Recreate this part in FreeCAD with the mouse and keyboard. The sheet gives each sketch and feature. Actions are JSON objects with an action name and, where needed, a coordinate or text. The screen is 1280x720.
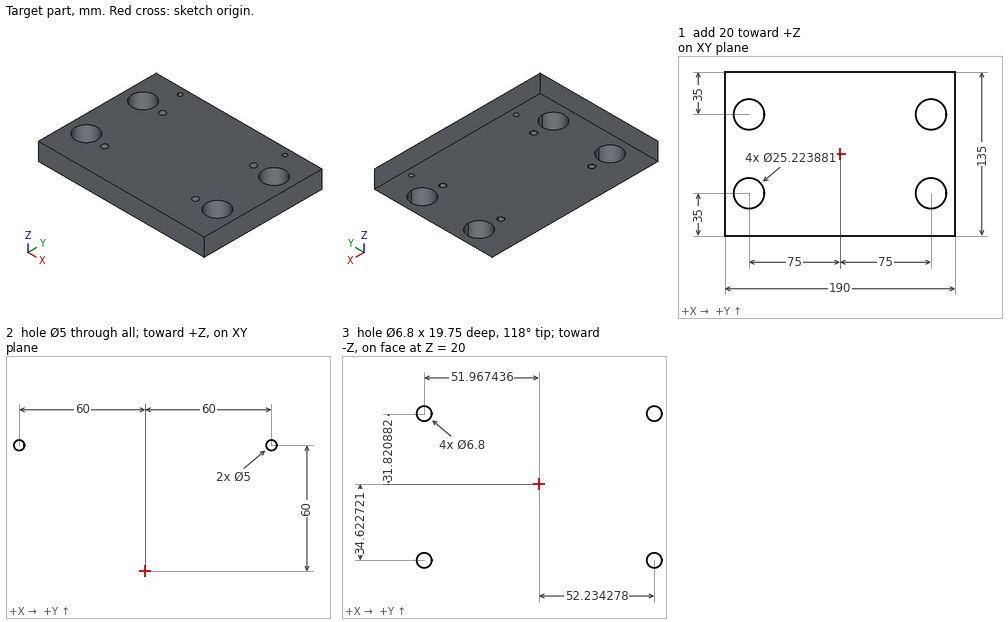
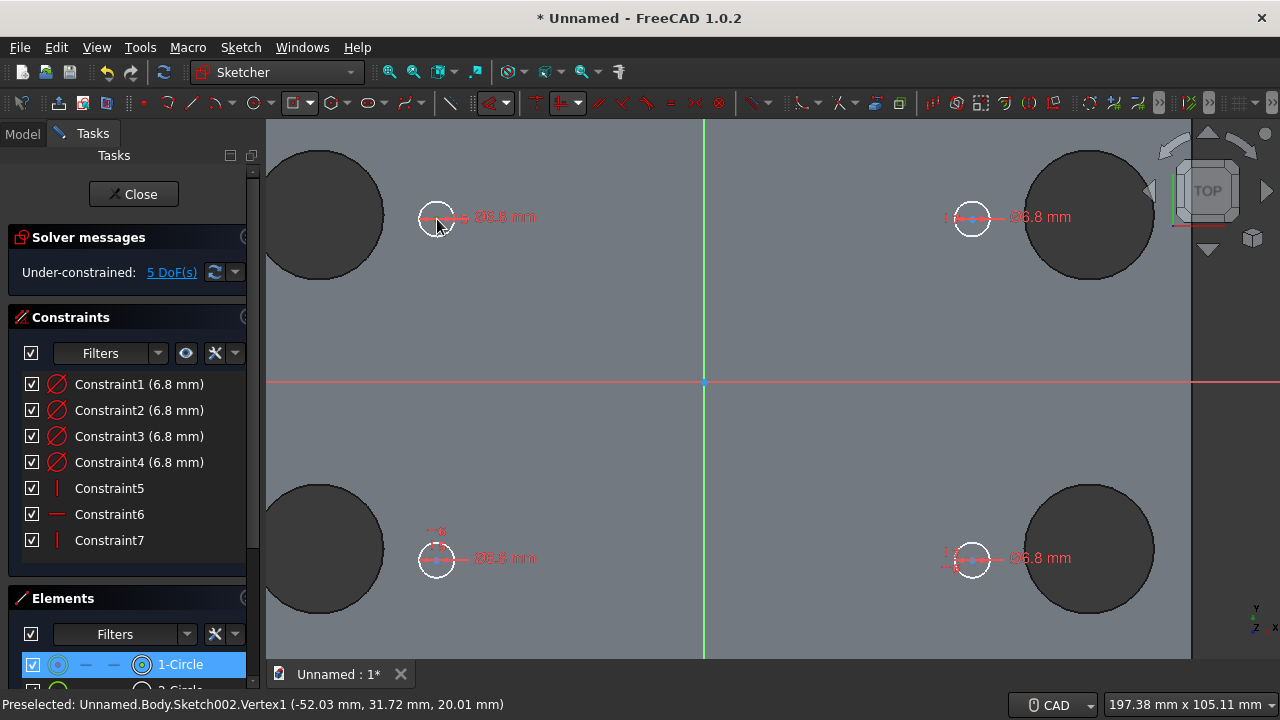
{"action": "left_click", "coordinate": [972, 219]}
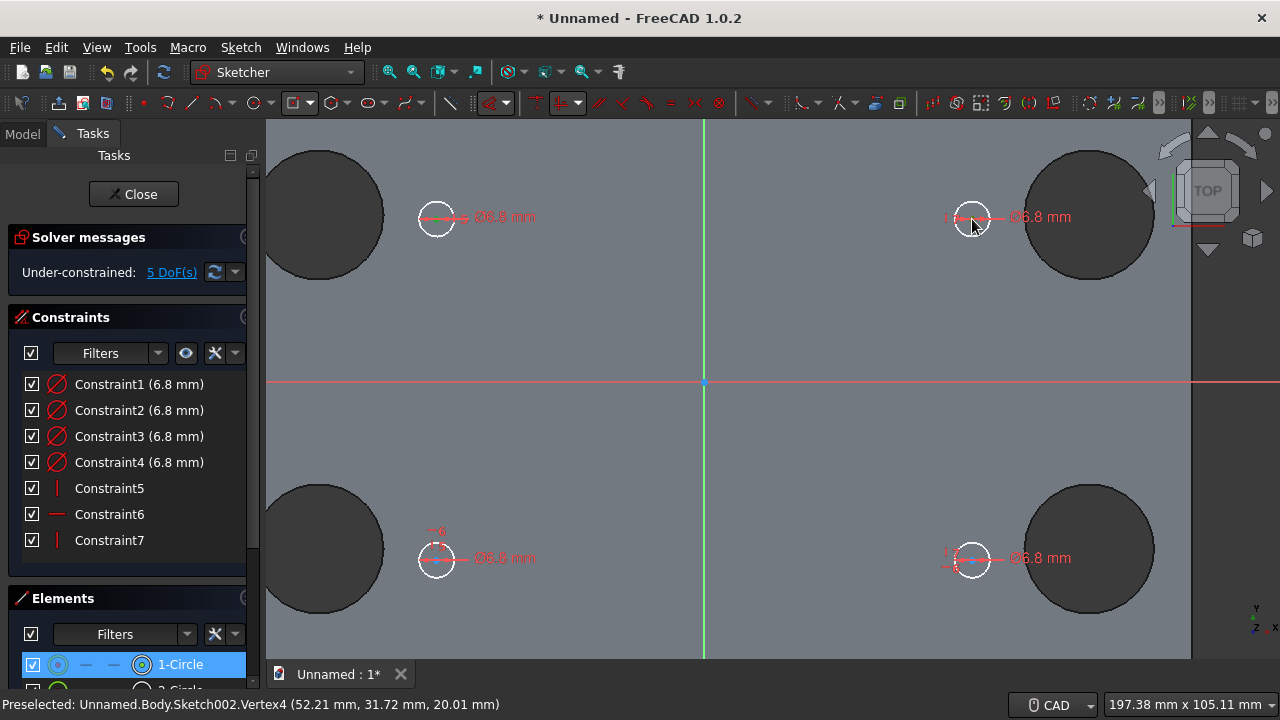
{"action": "key", "text": "h"}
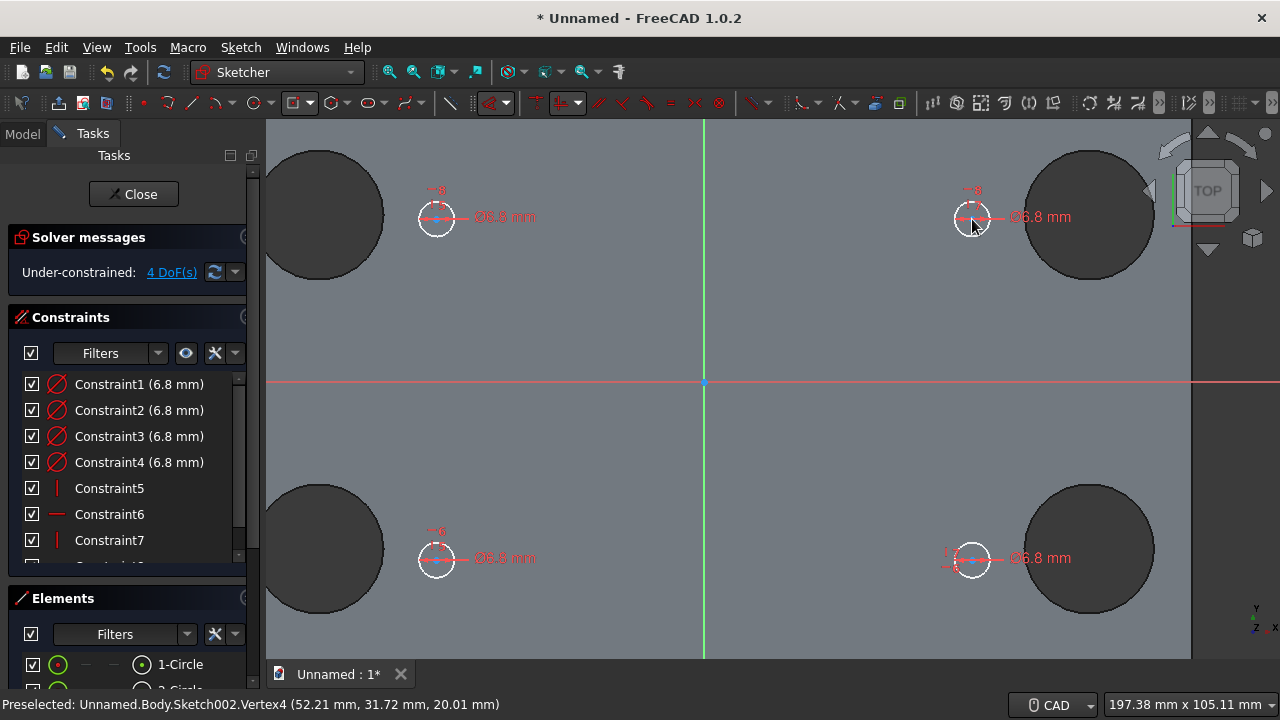
{"action": "left_click", "coordinate": [437, 219]}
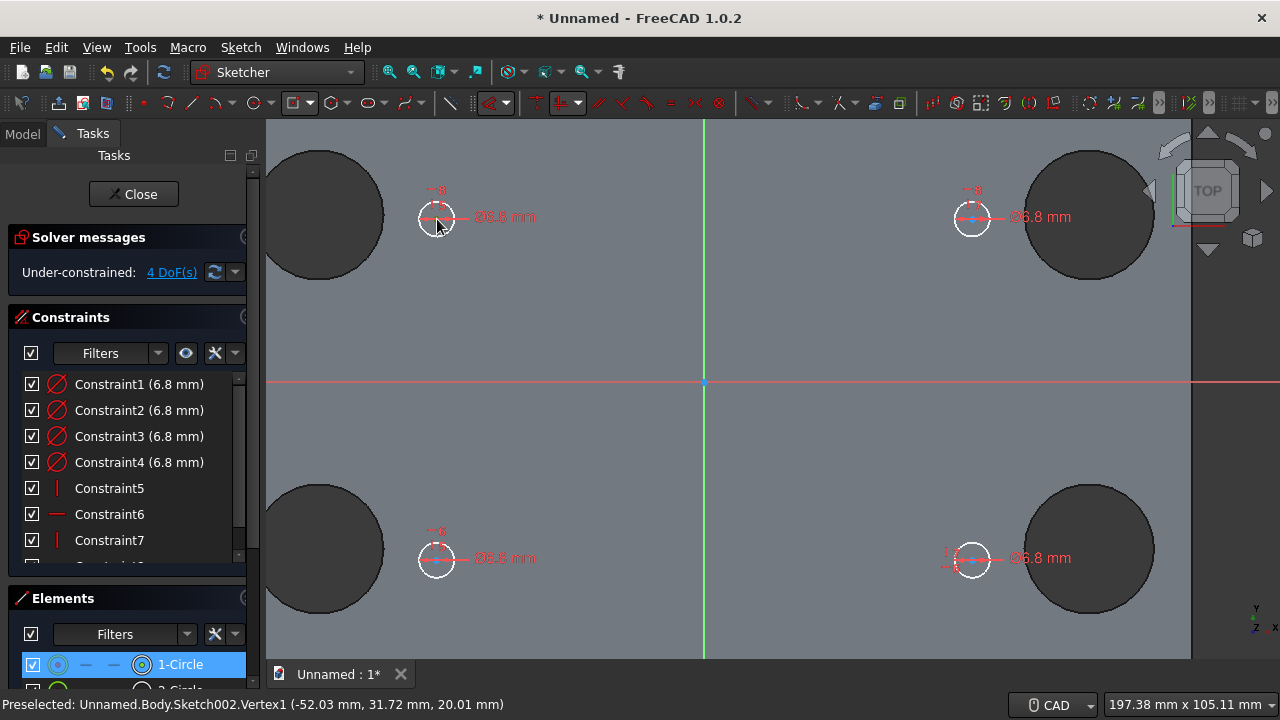
{"action": "left_click", "coordinate": [508, 104]}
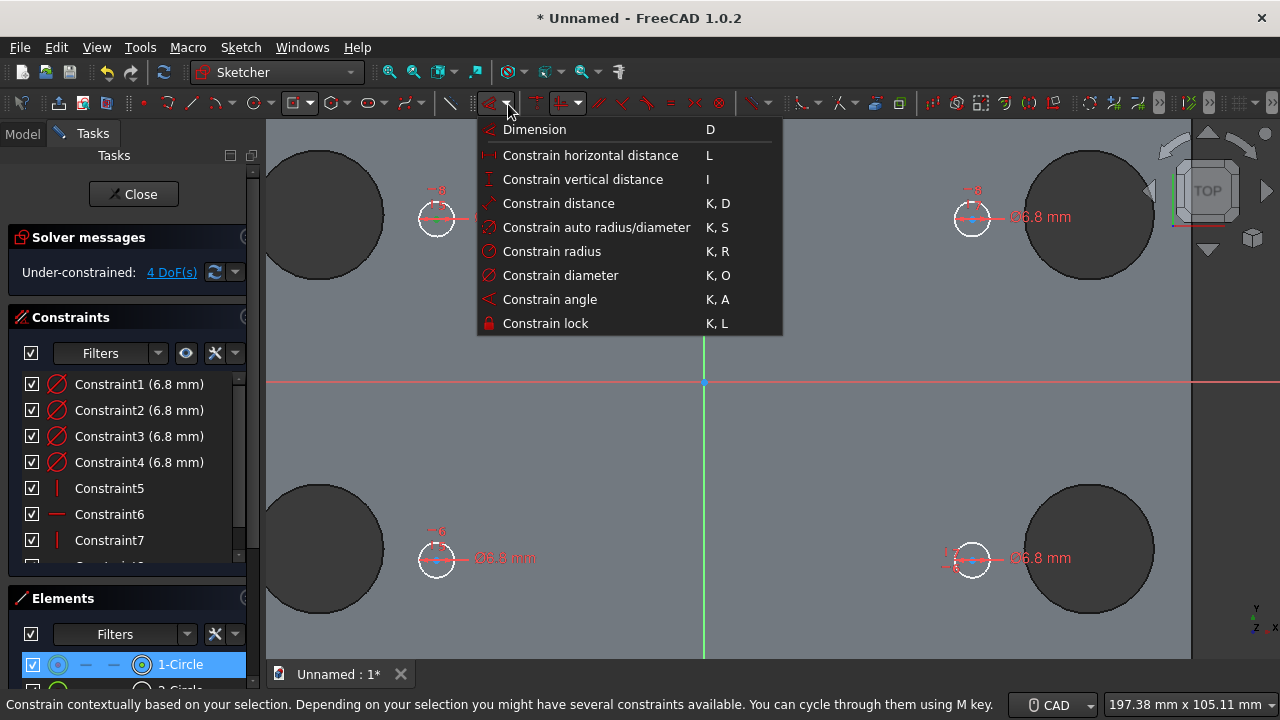
{"action": "left_click", "coordinate": [630, 155]}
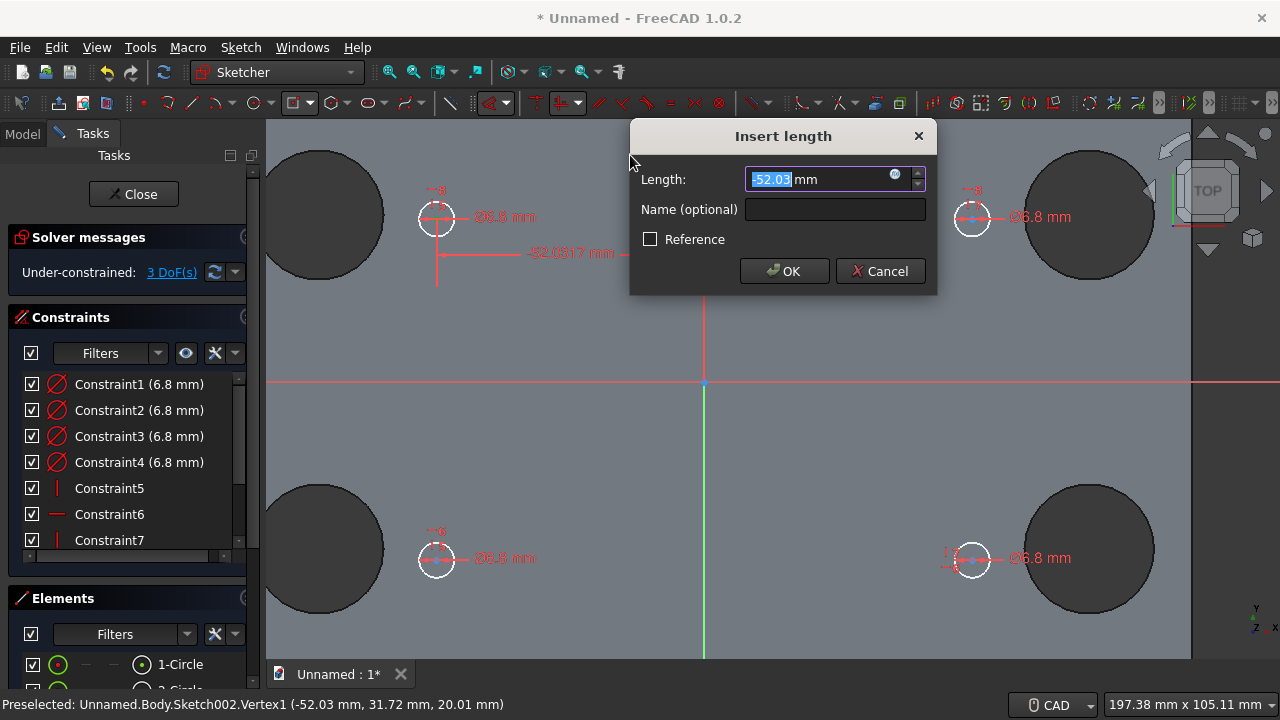
{"action": "type", "text": "-51.967436"}
{"action": "key", "text": "Return"}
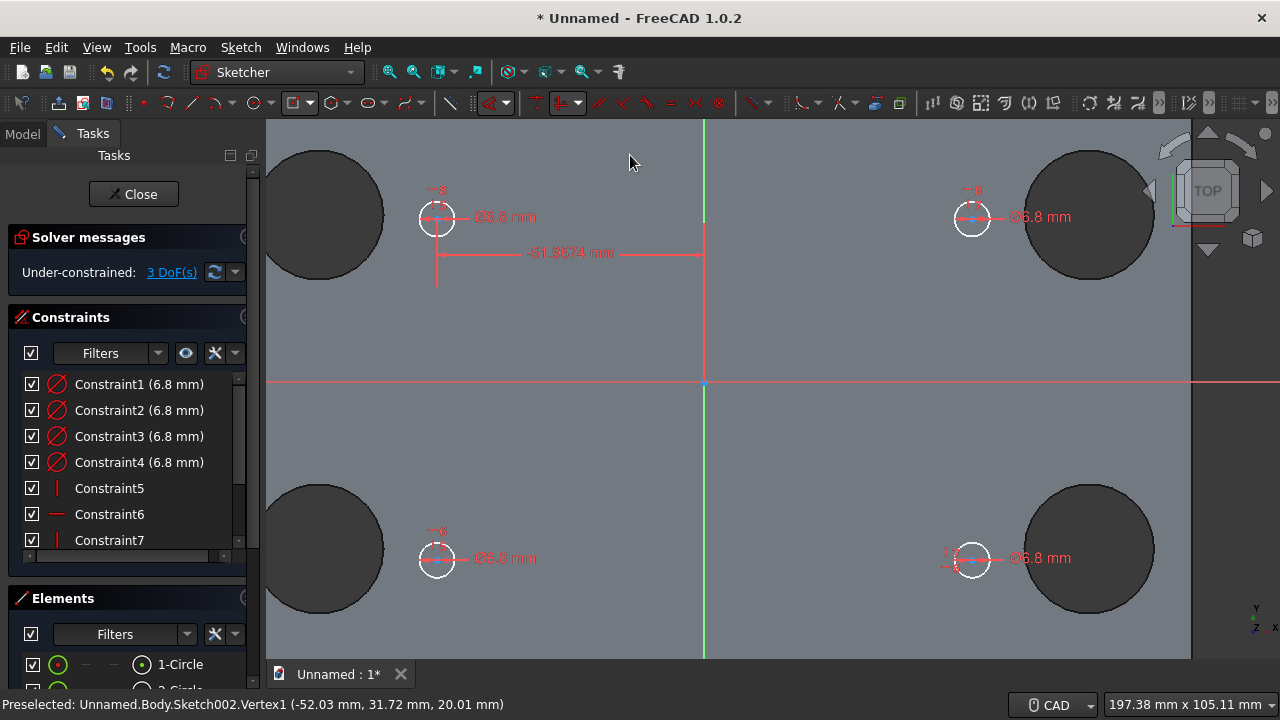
{"action": "left_click", "coordinate": [437, 219]}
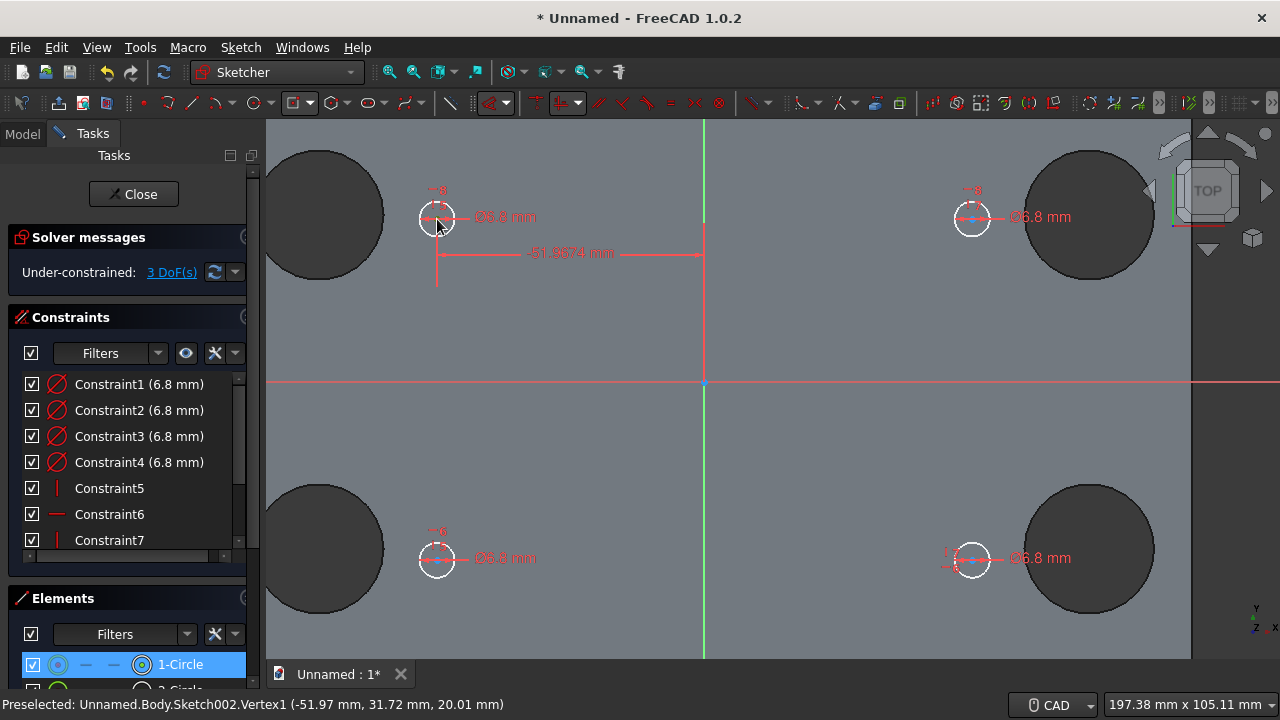
{"action": "left_click", "coordinate": [508, 104]}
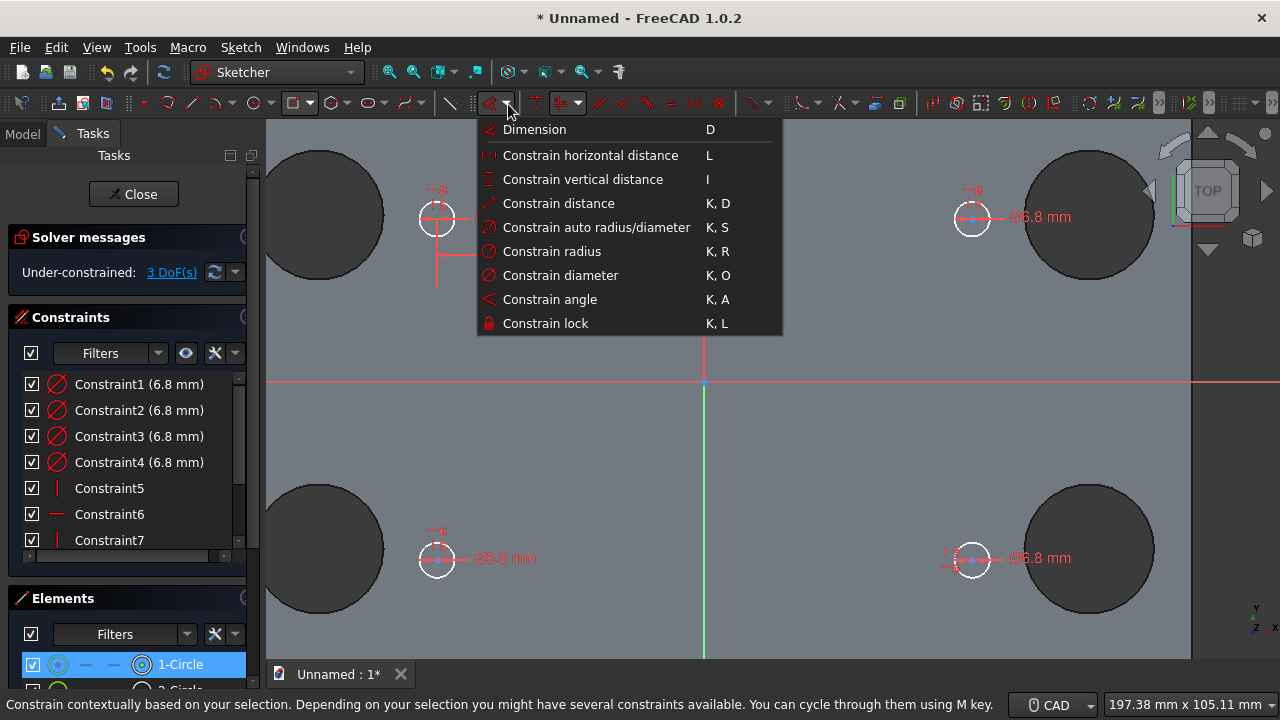
{"action": "left_click", "coordinate": [630, 179]}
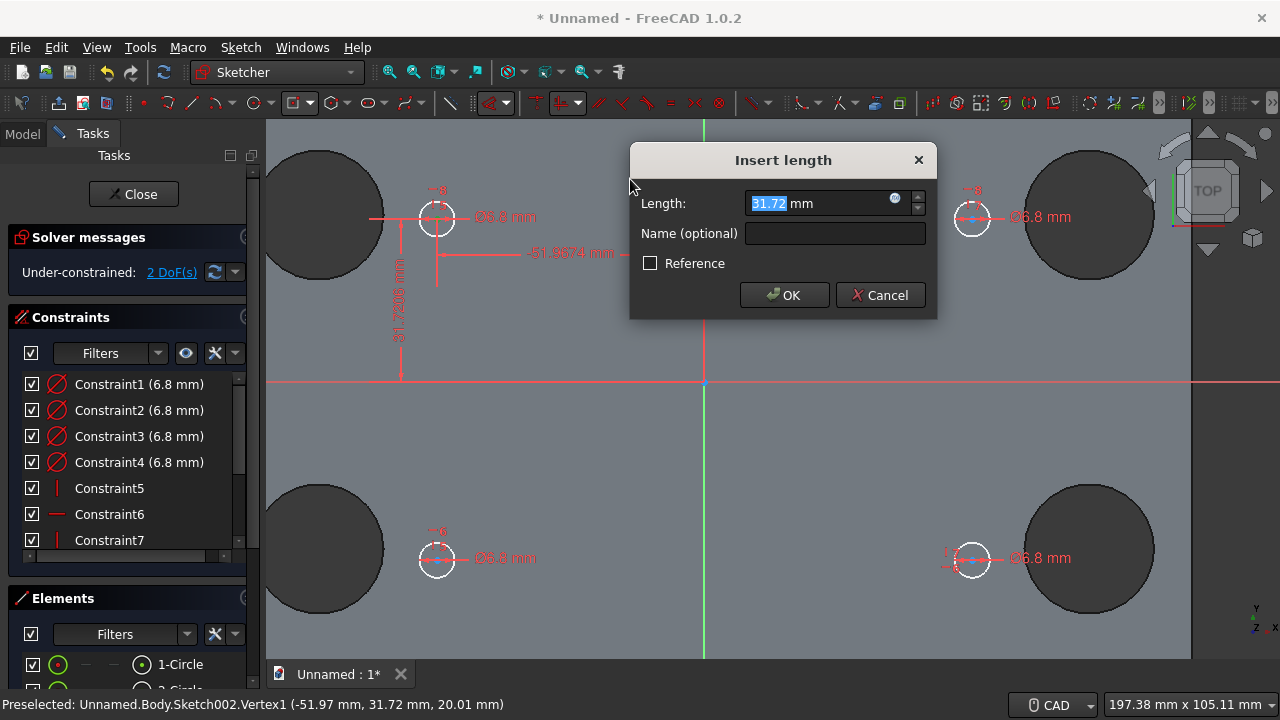
{"action": "type", "text": "31.820882"}
{"action": "key", "text": "Return"}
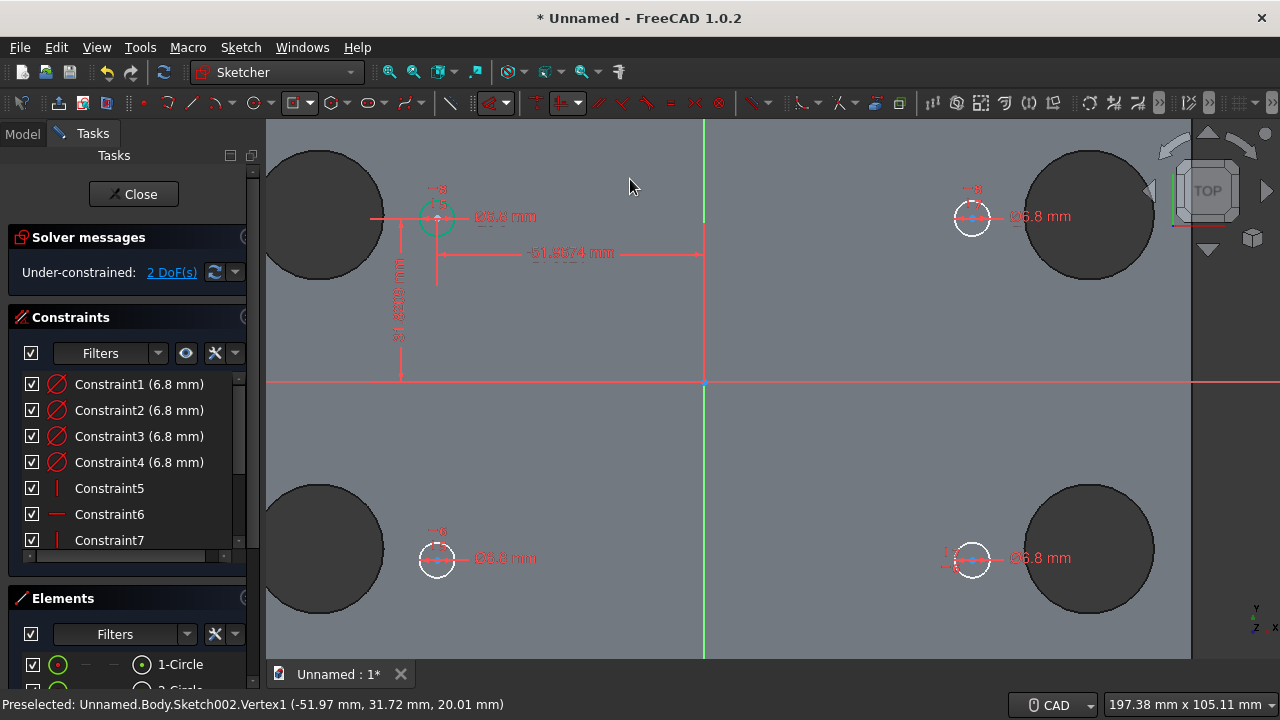
{"action": "left_click", "coordinate": [437, 560]}